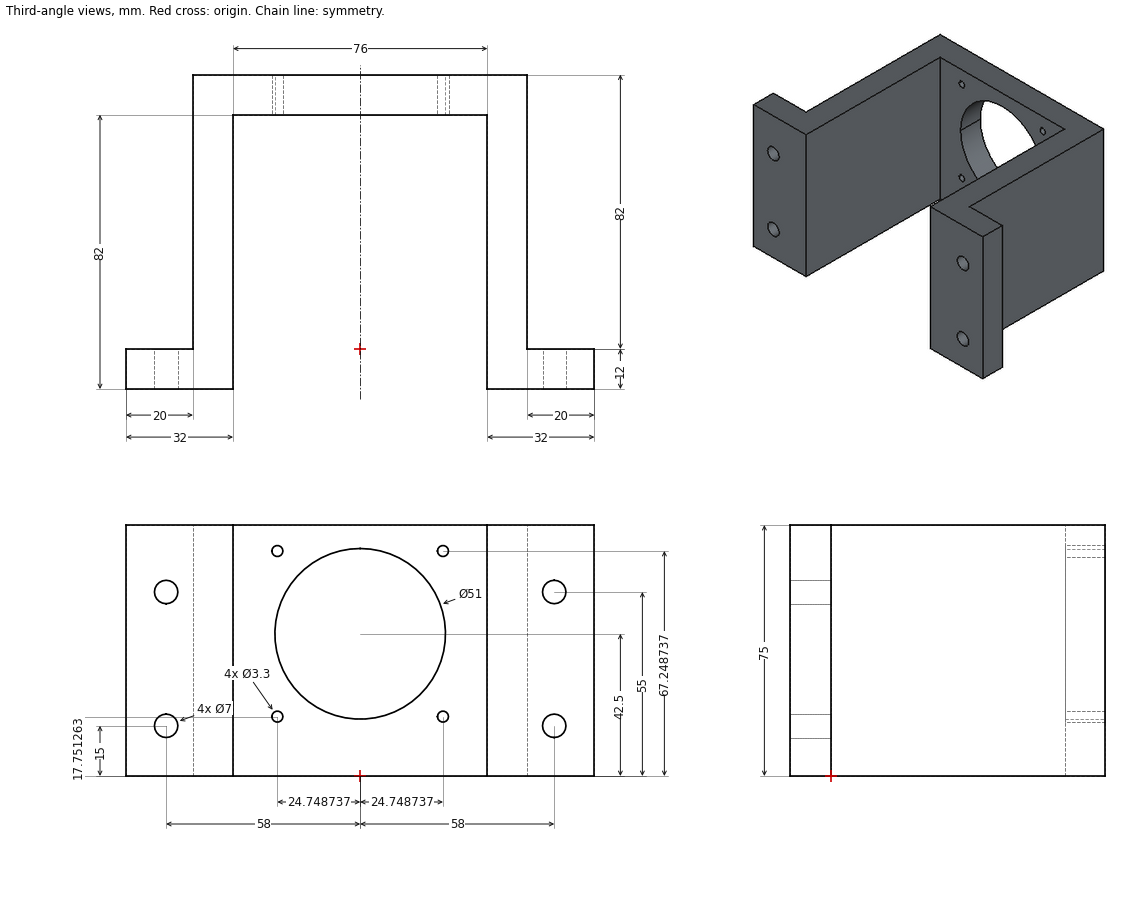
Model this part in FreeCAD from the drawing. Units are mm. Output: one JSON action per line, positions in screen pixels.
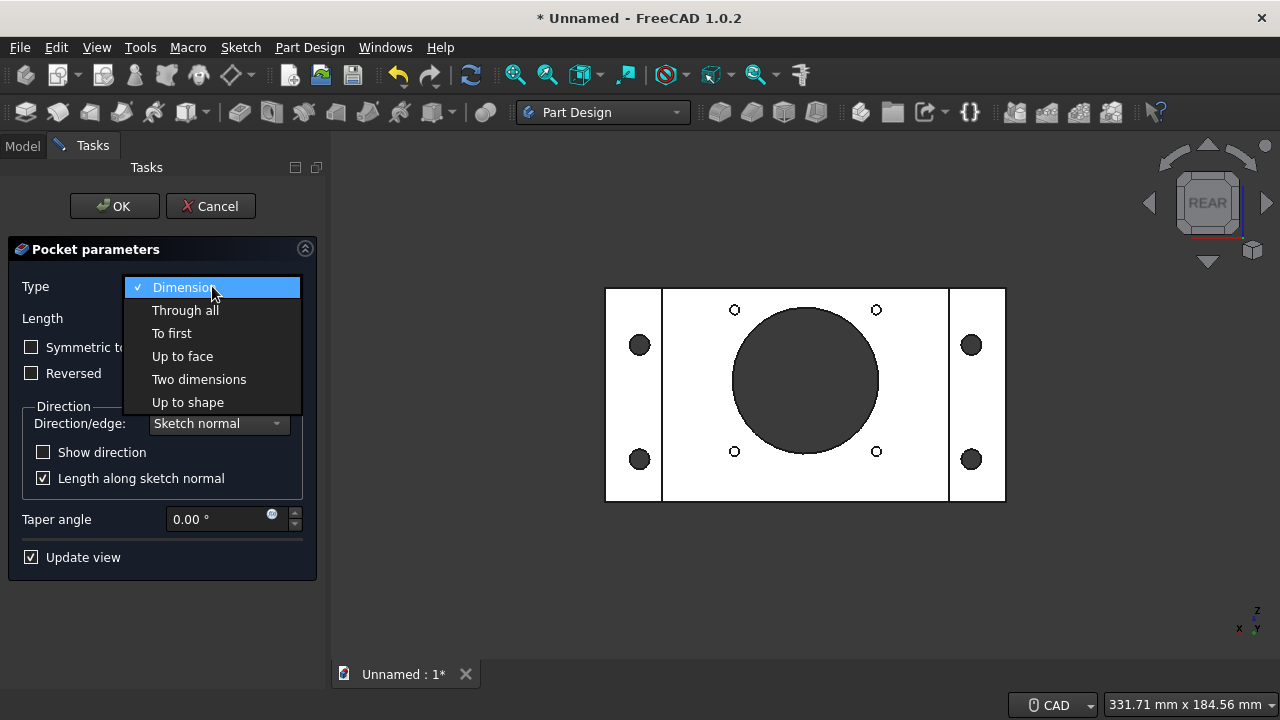
{"action": "left_click", "coordinate": [212, 310]}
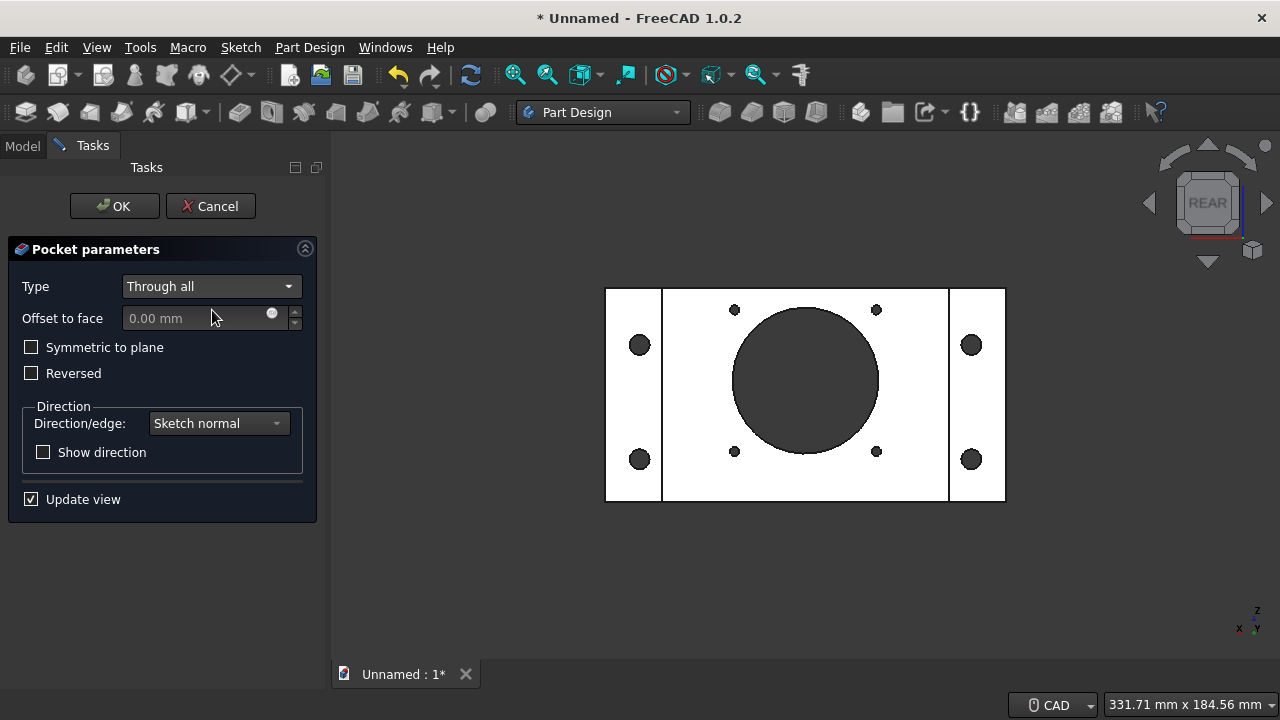
{"action": "left_click", "coordinate": [115, 206]}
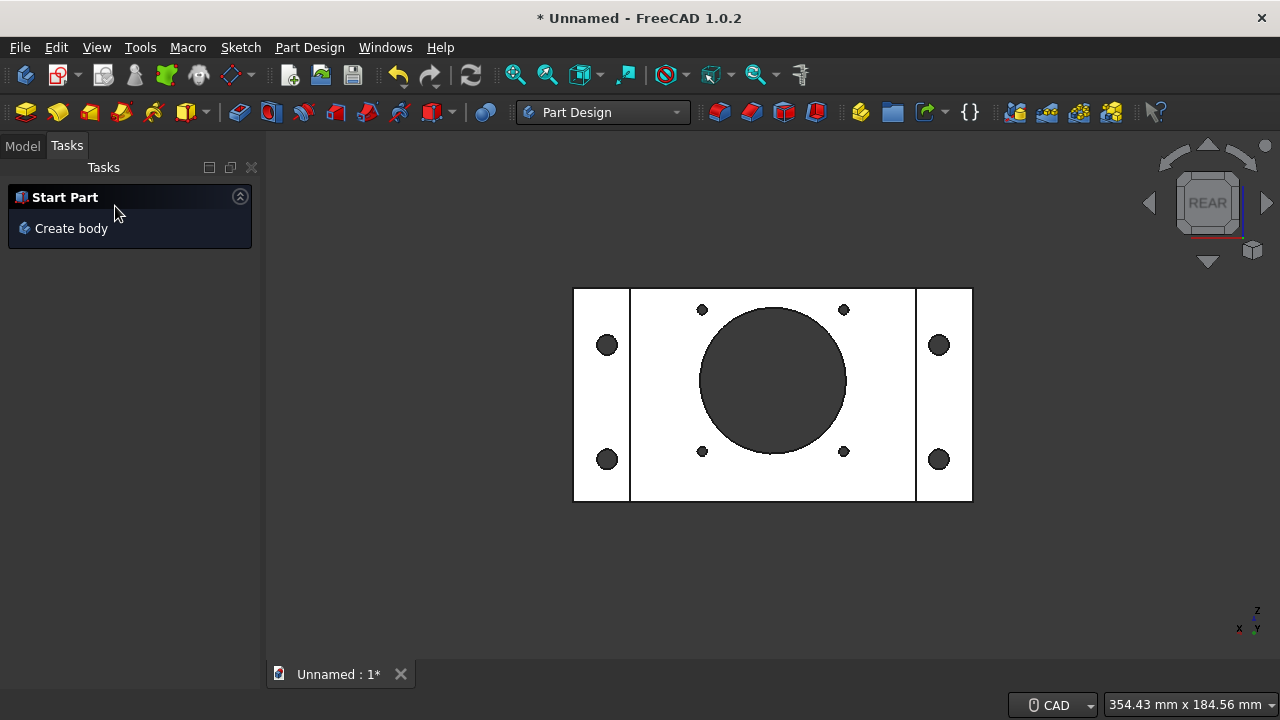
{"action": "key", "text": "0"}